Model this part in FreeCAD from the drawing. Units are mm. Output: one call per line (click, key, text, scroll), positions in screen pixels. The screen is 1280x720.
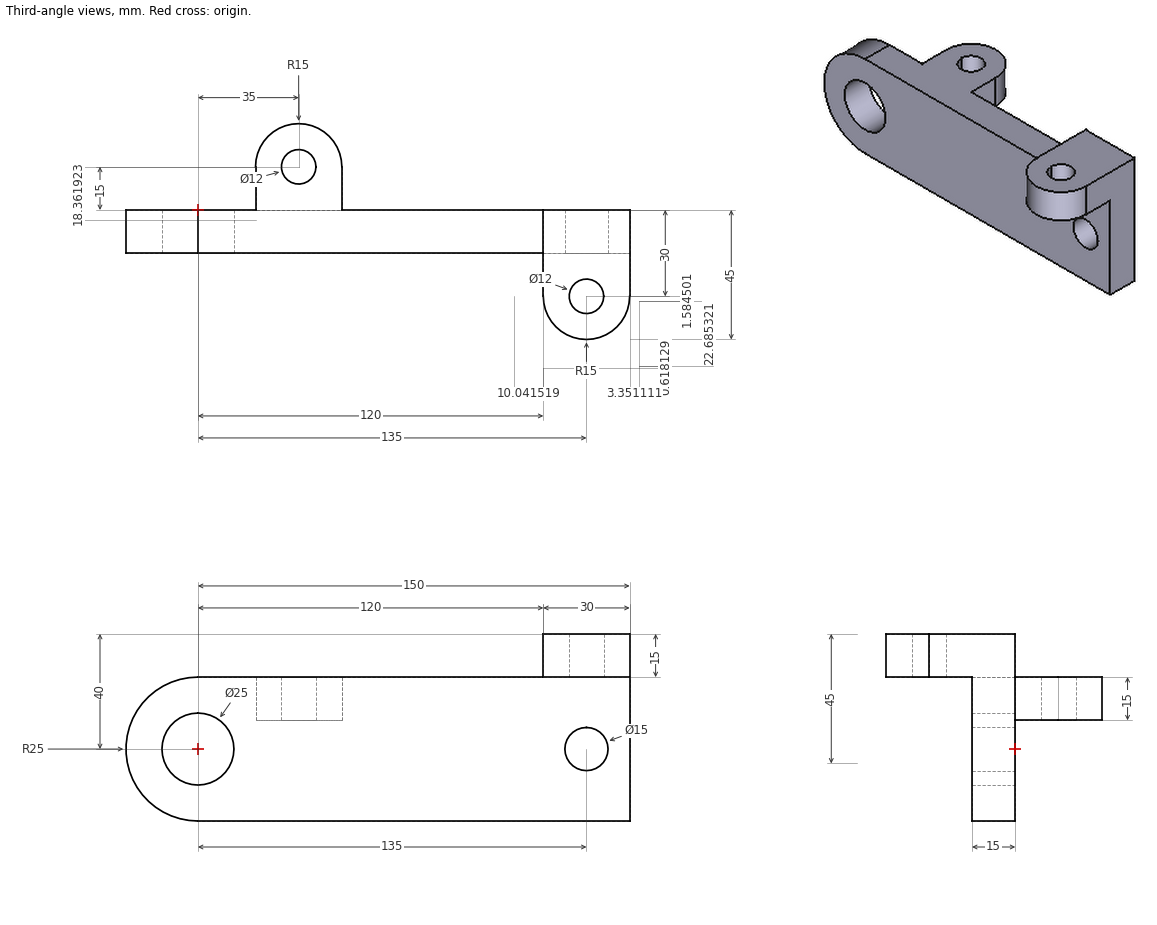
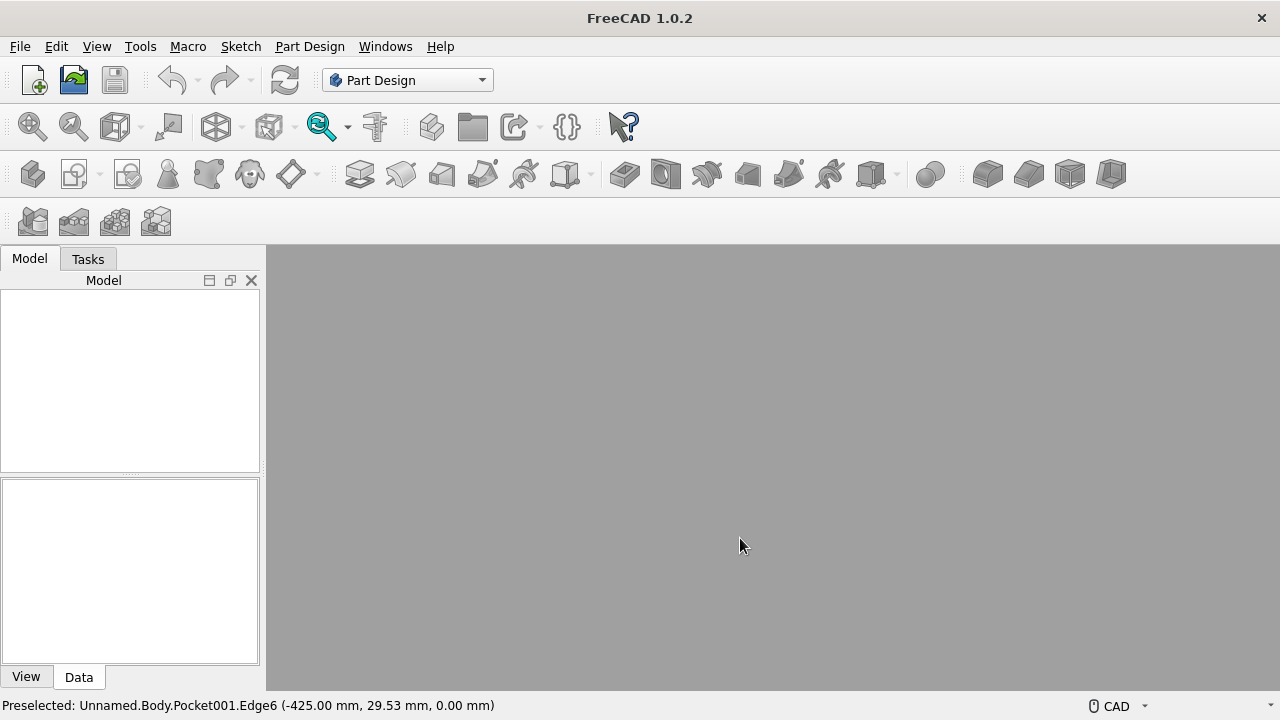
click(33, 80)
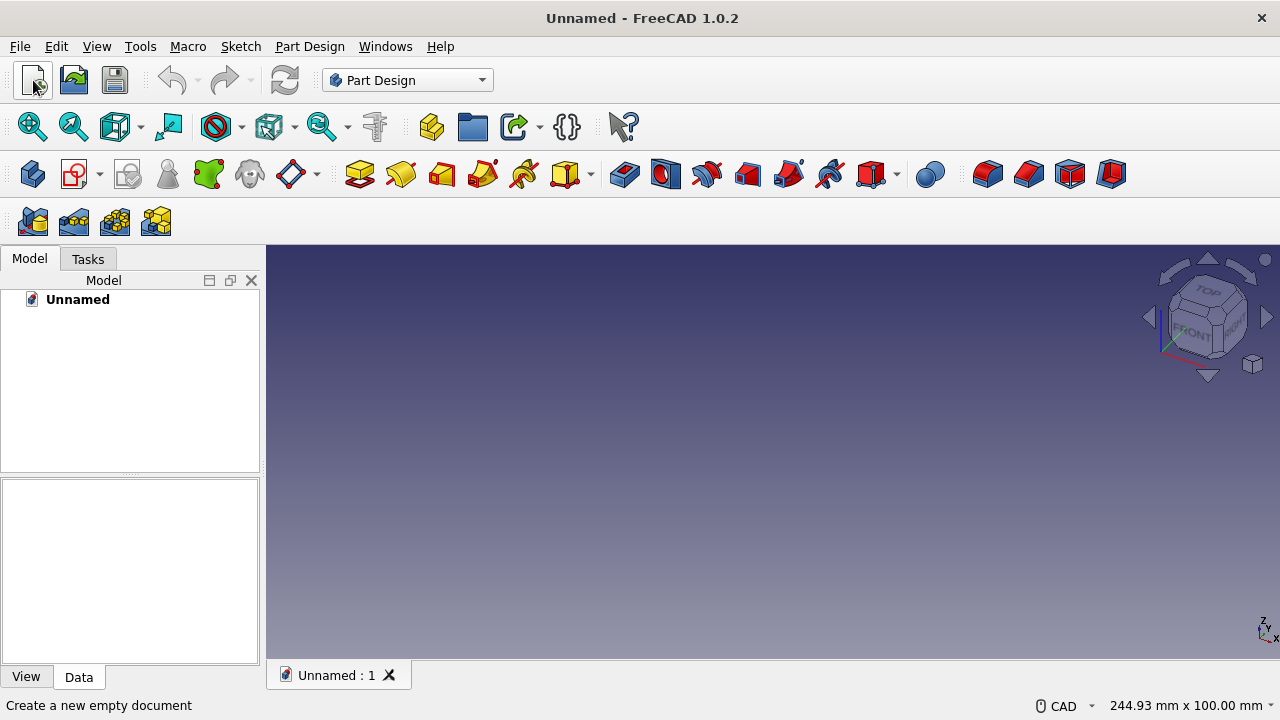
click(74, 174)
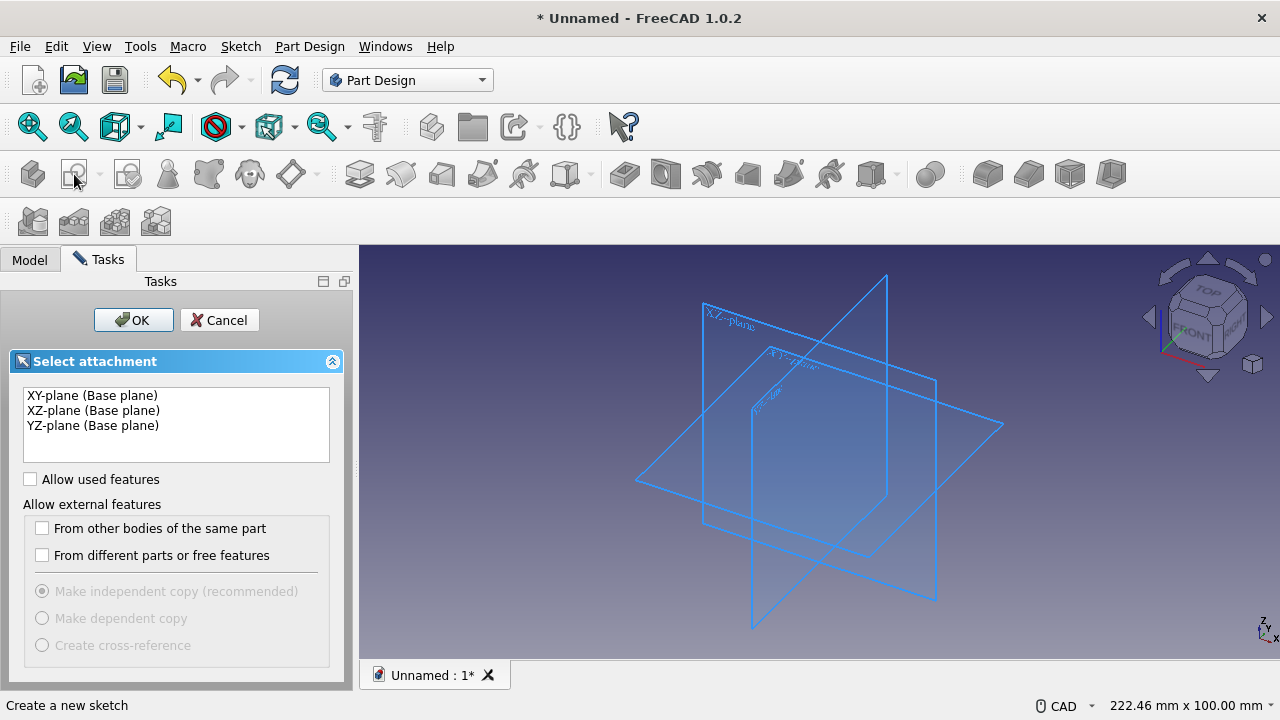
click(84, 410)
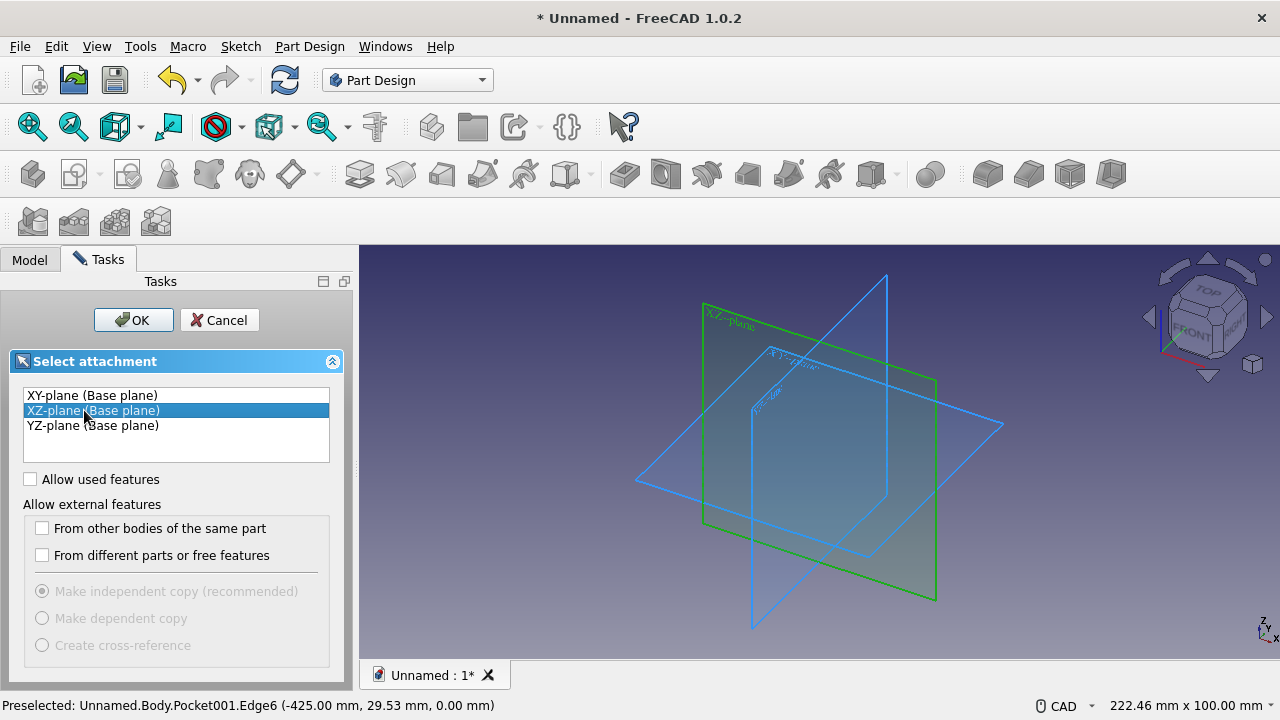
click(134, 320)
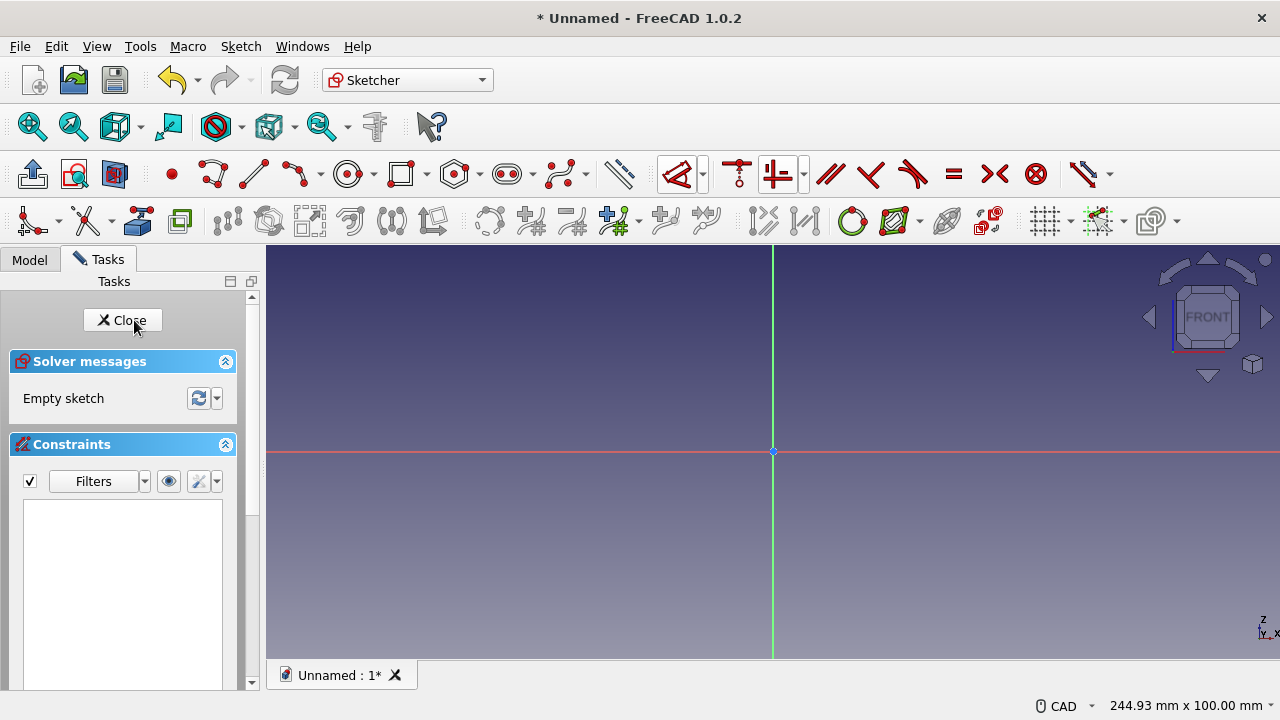
scroll(294, 452, down, 2)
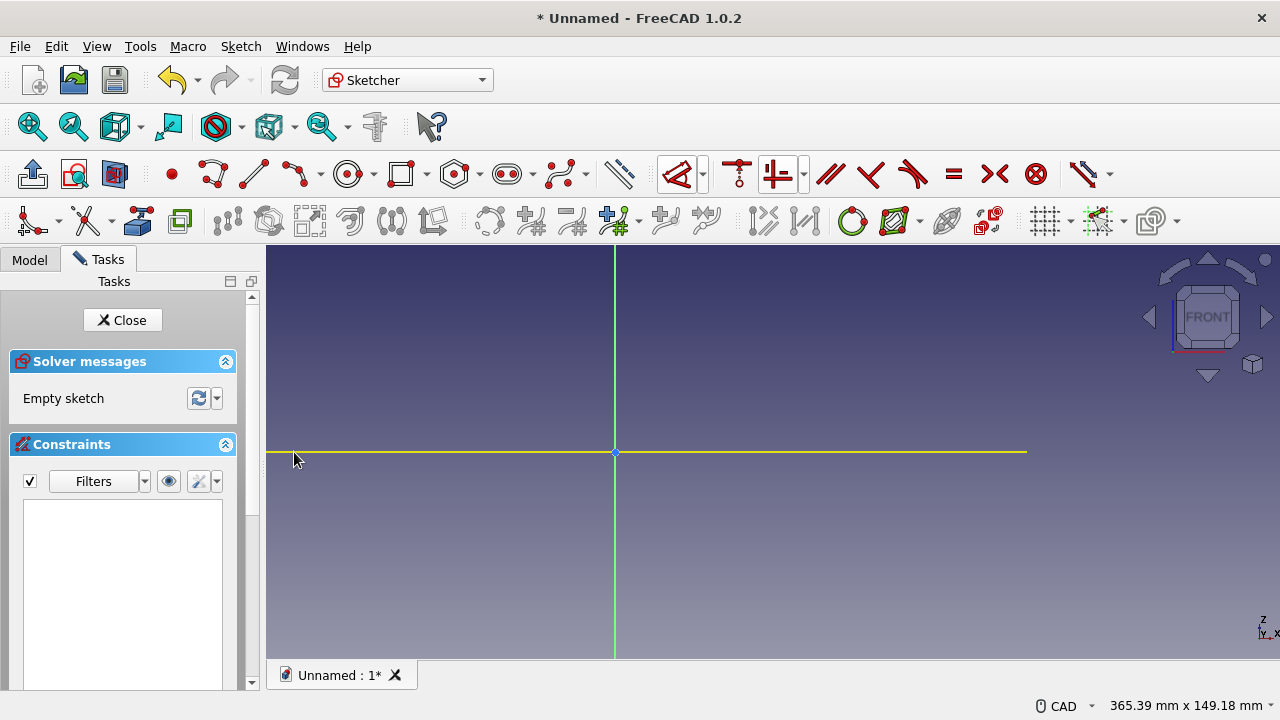
click(213, 174)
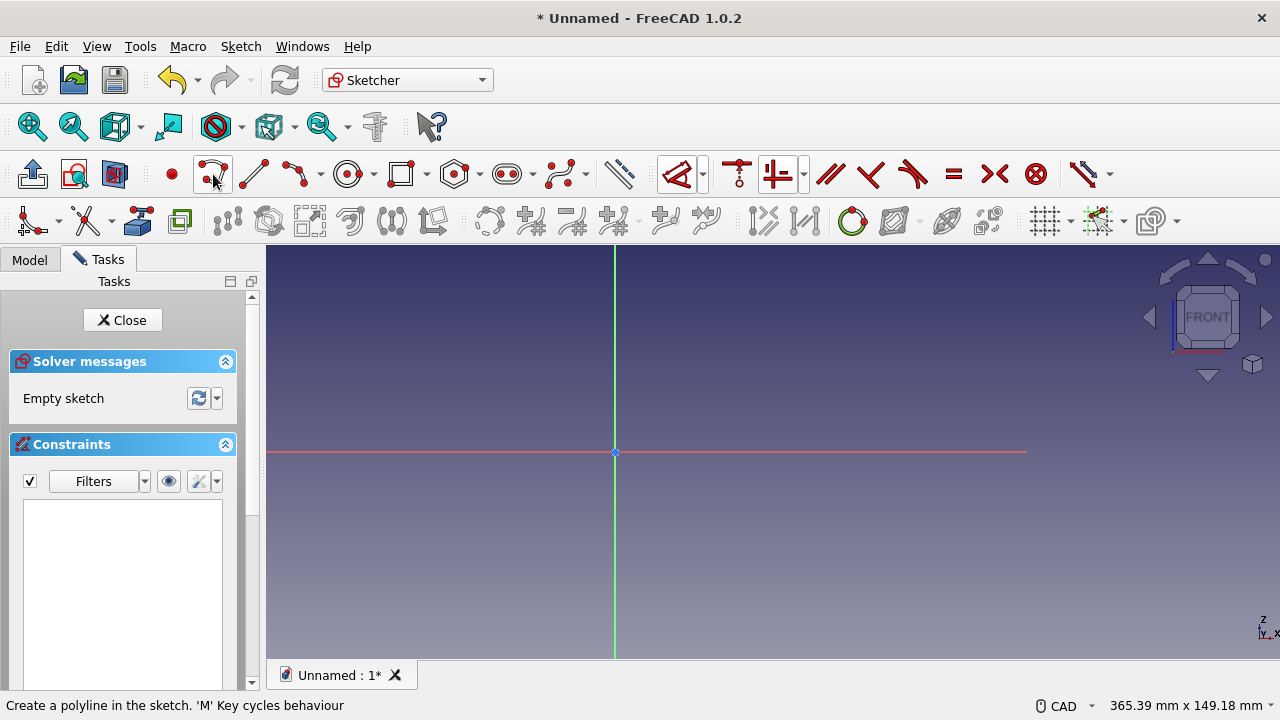
click(615, 383)
click(1031, 383)
click(1031, 522)
click(615, 522)
right_click(615, 522)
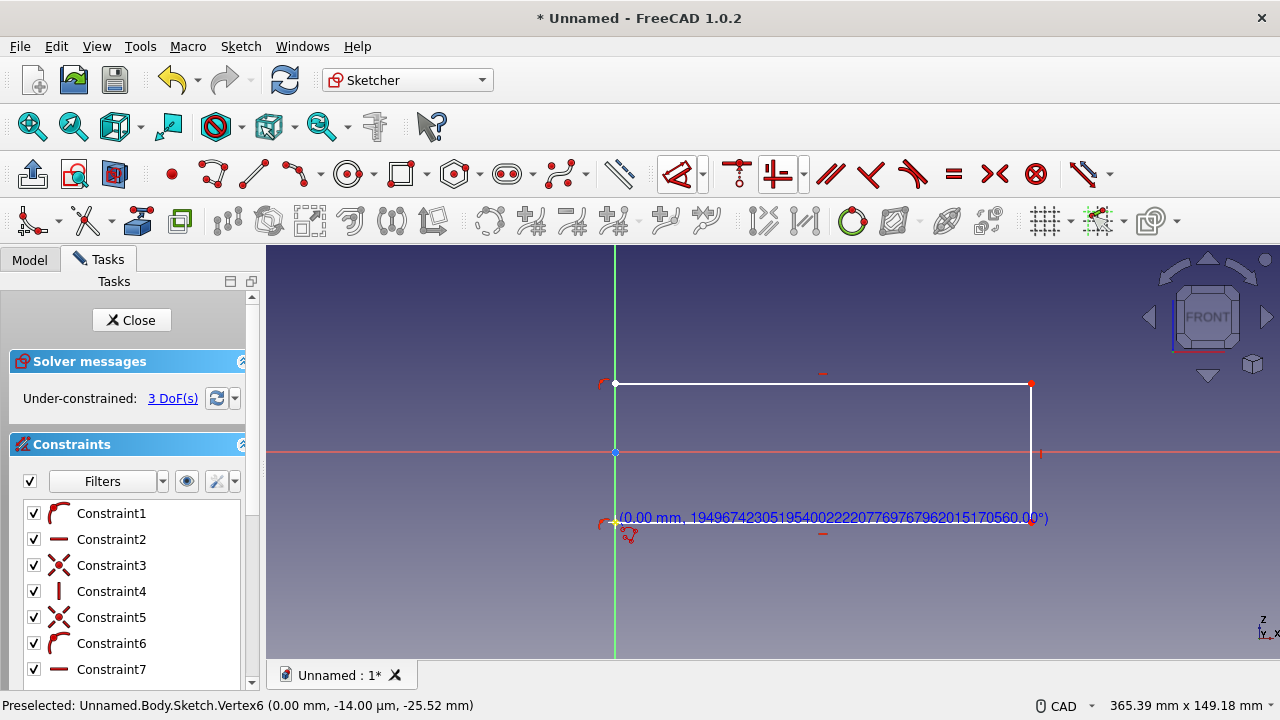
click(294, 174)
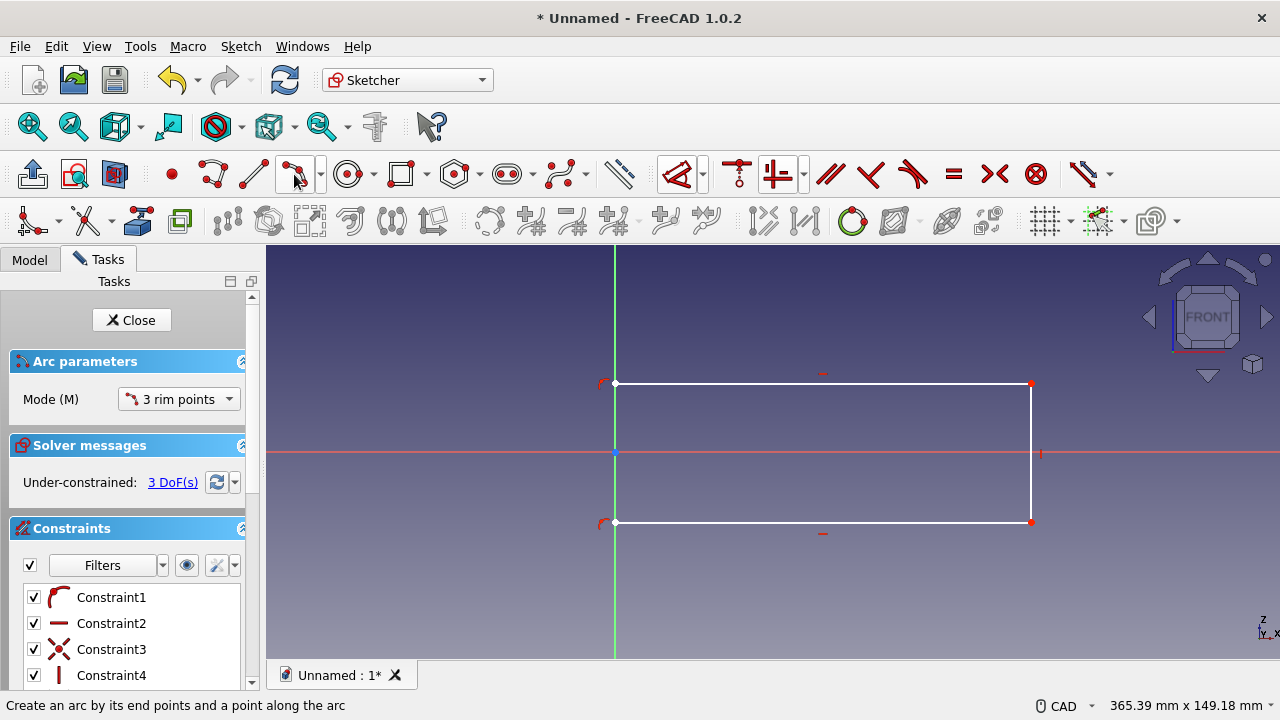
click(615, 523)
click(615, 384)
click(549, 431)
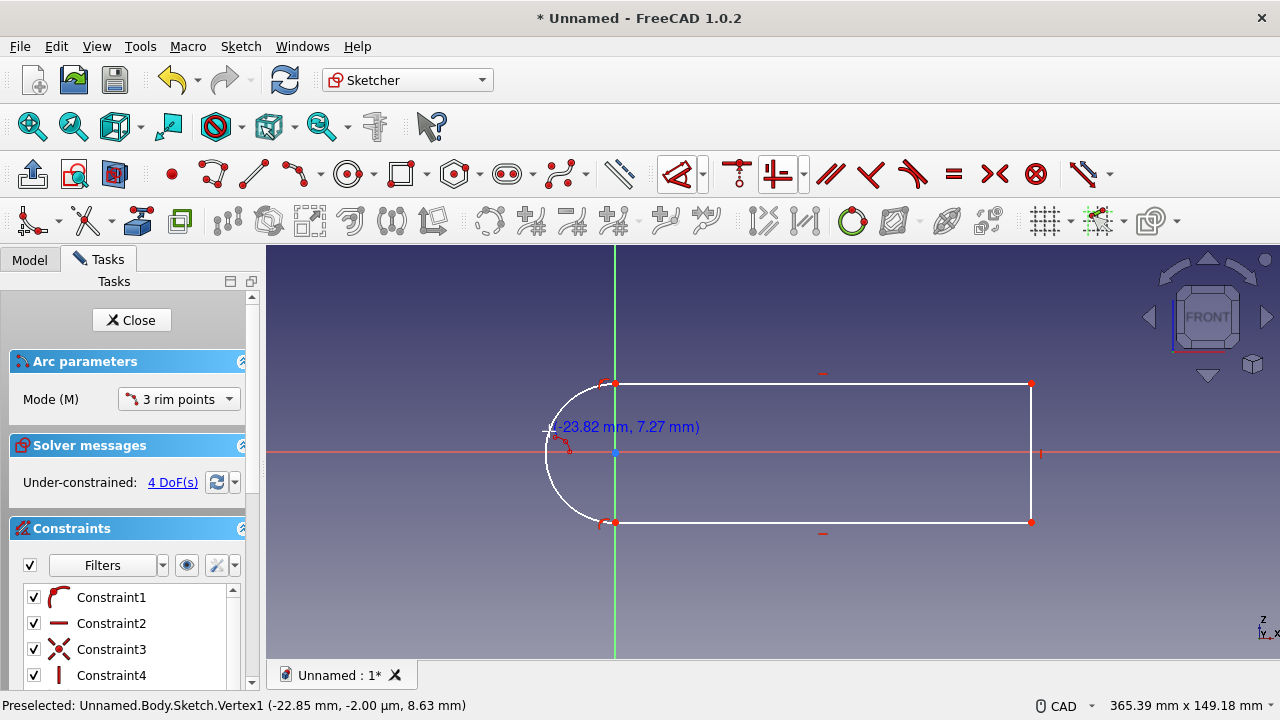
click(348, 174)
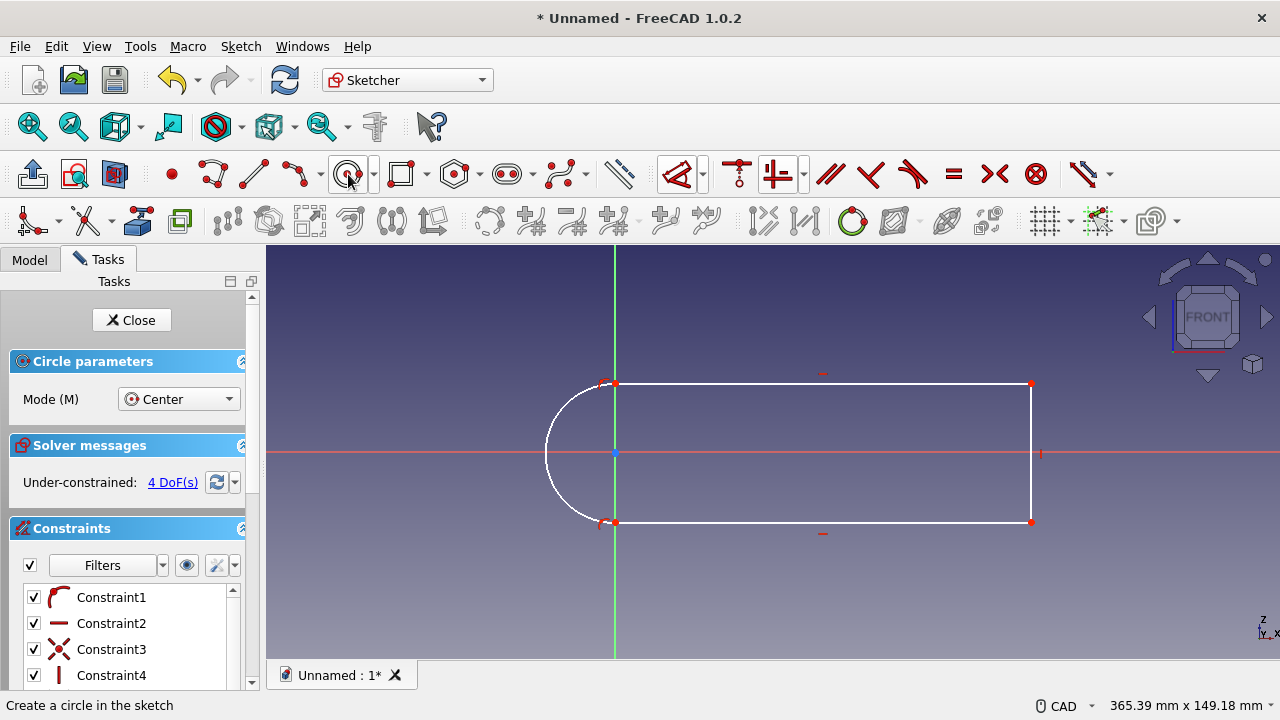
click(615, 452)
click(640, 428)